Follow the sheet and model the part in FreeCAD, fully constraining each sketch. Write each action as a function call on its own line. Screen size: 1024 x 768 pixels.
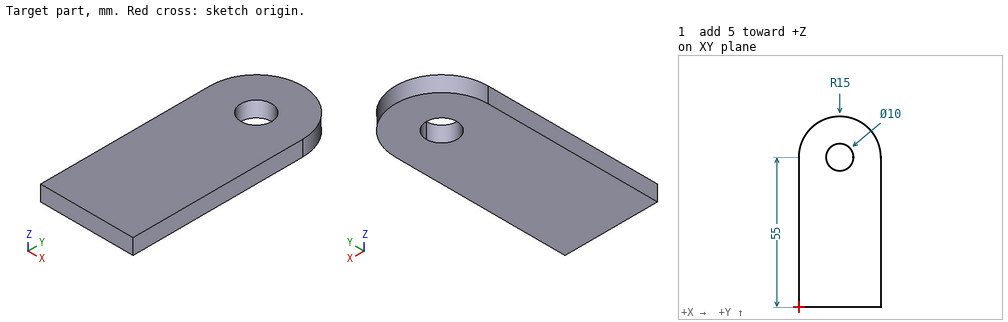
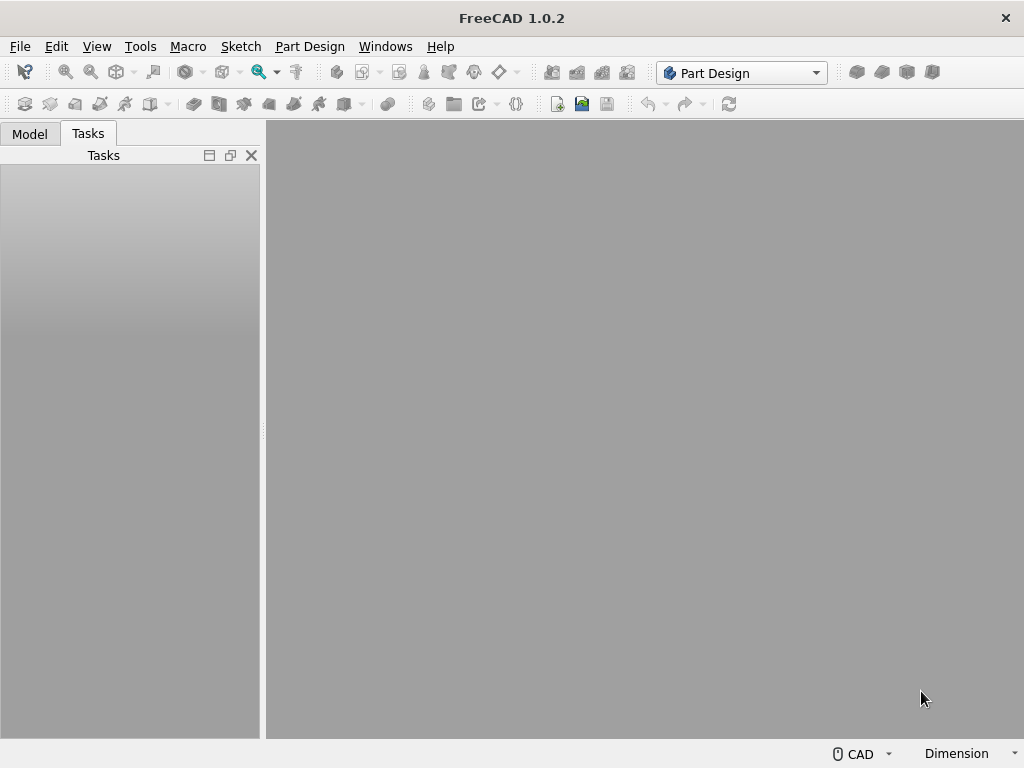
click(557, 104)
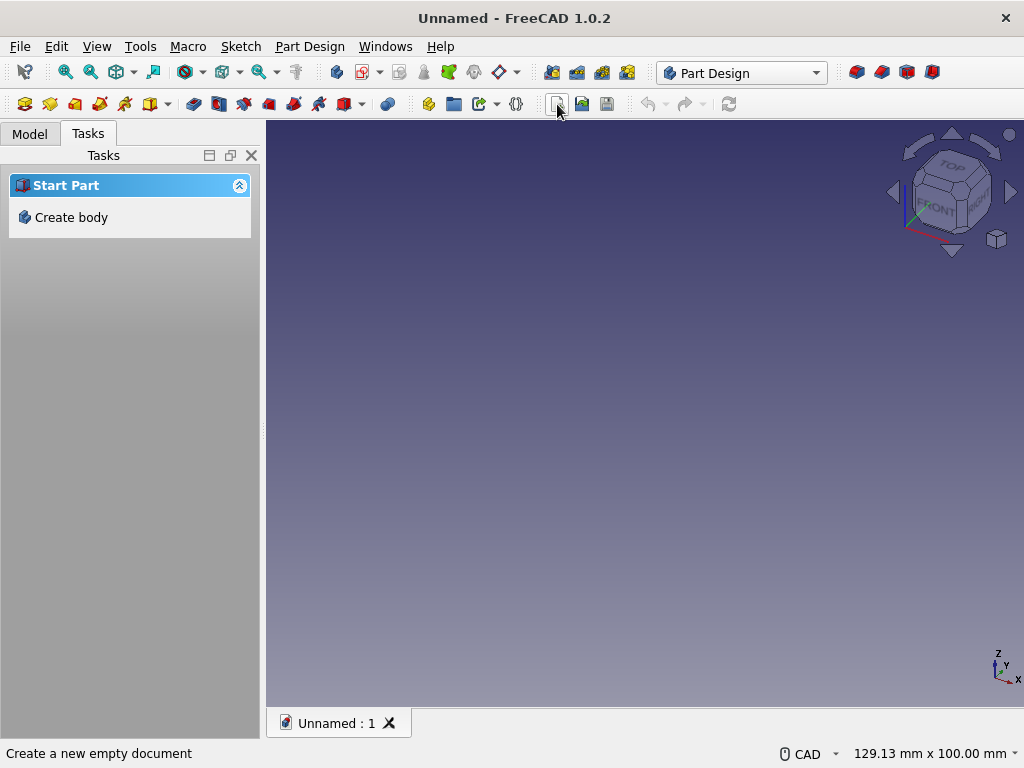
click(362, 72)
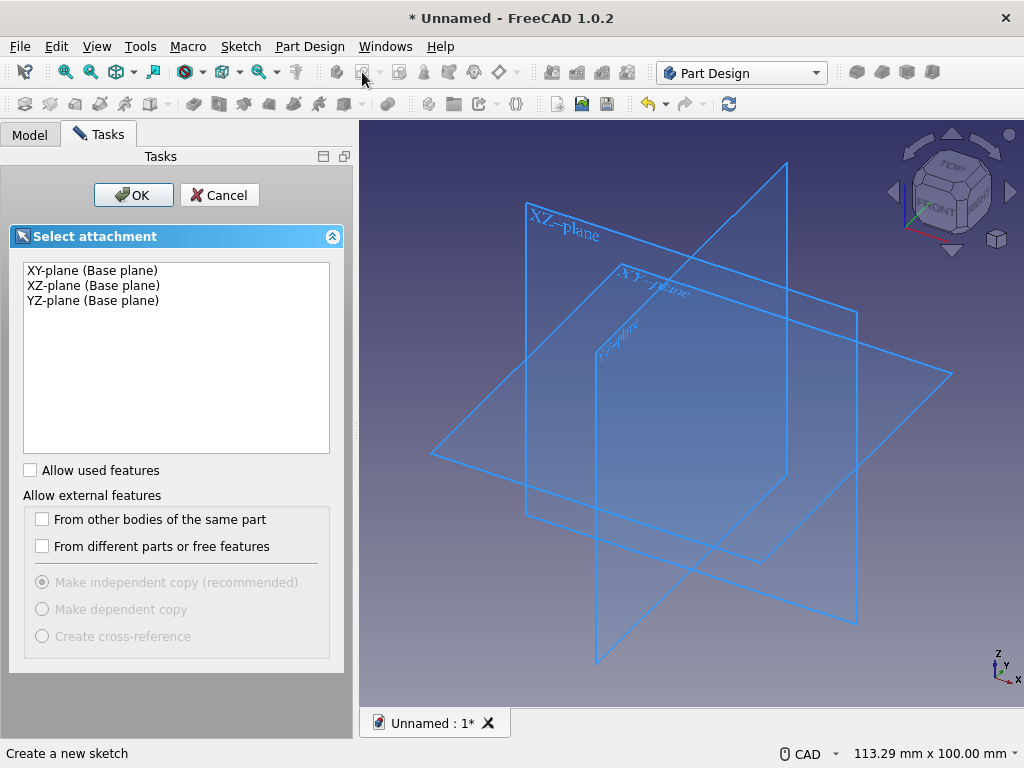
click(84, 270)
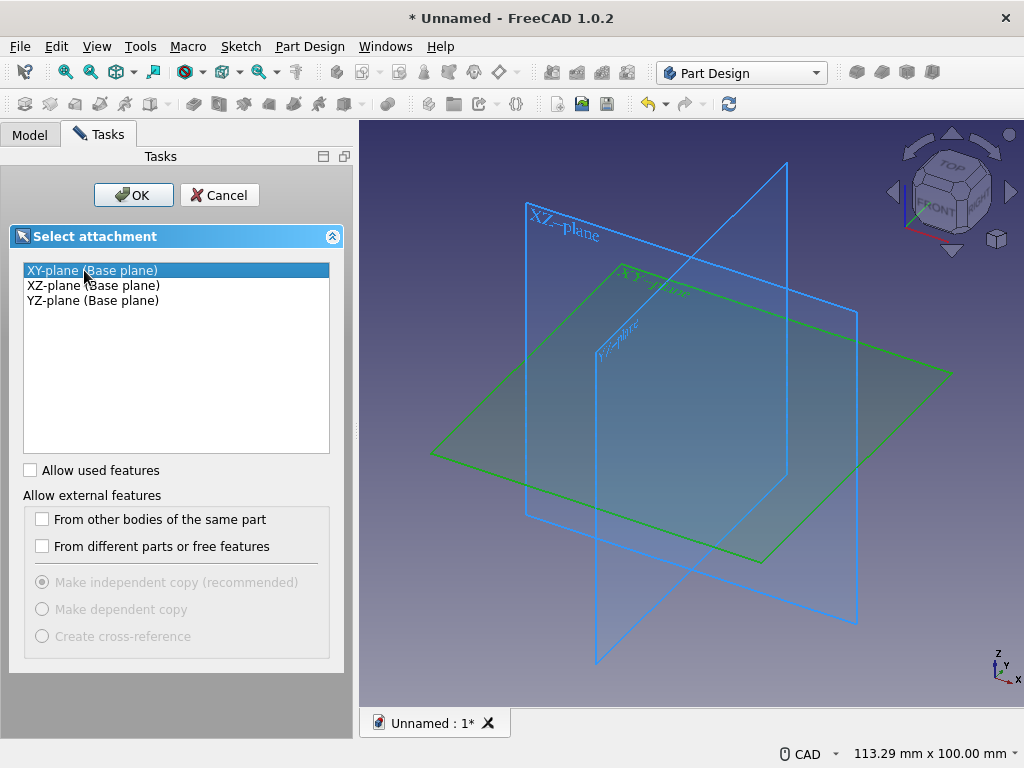
click(134, 195)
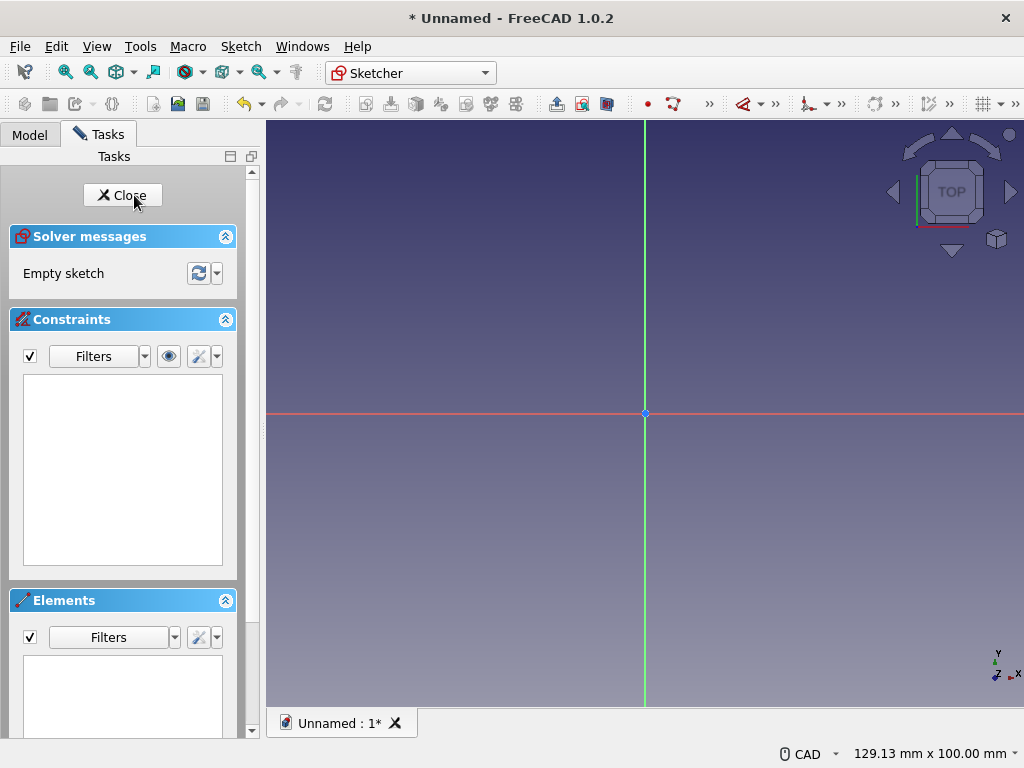
scroll(294, 679, down, 2)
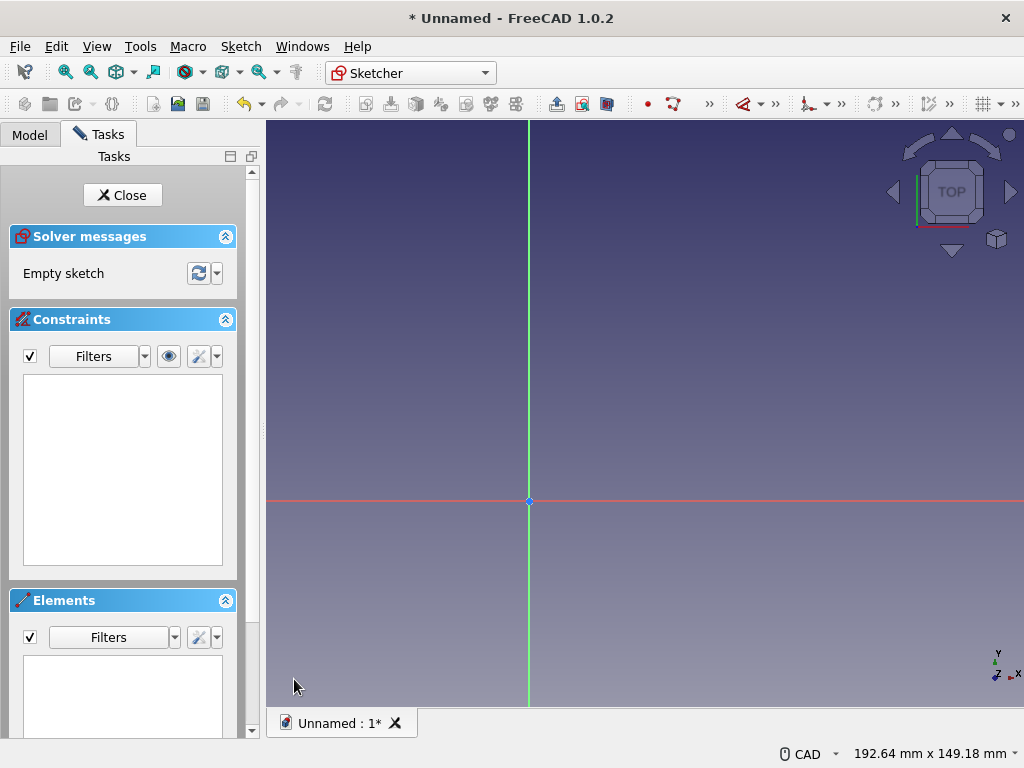
scroll(612, 262, up, 2)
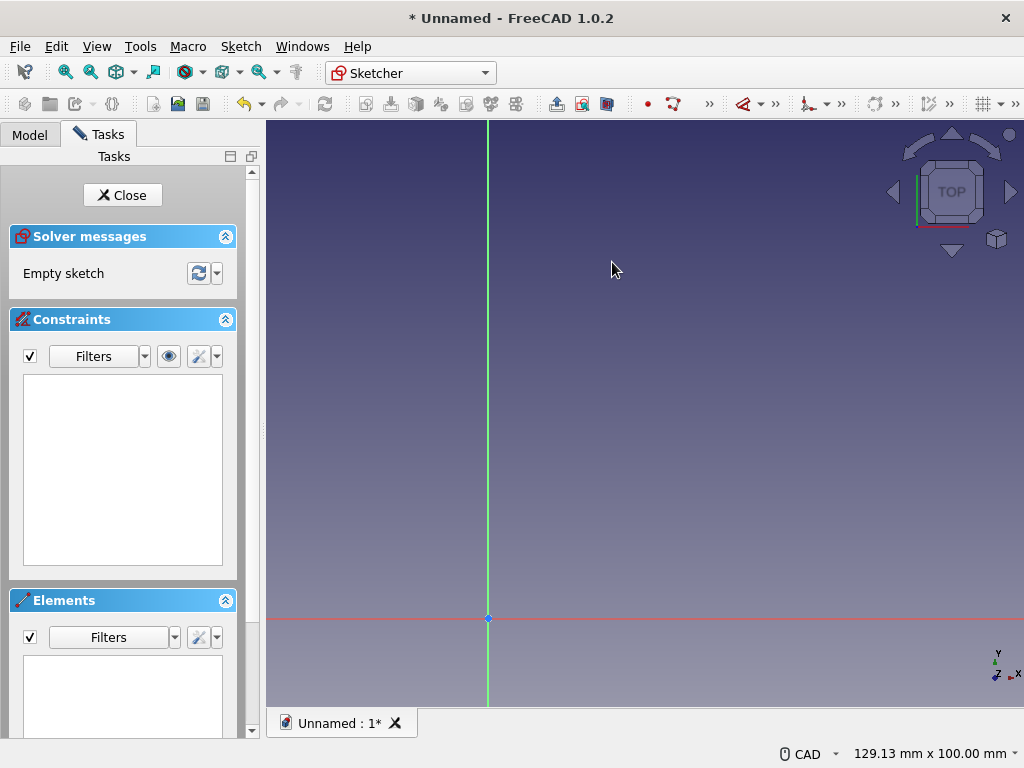
click(673, 104)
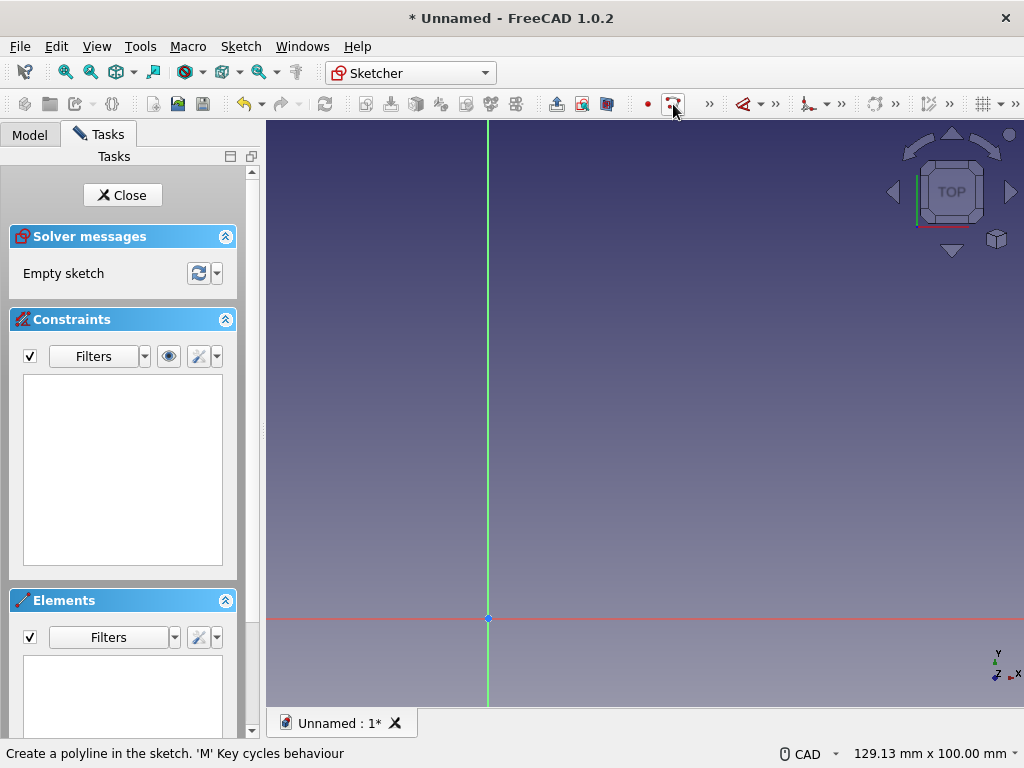
click(488, 296)
click(488, 619)
click(664, 610)
click(664, 296)
right_click(664, 296)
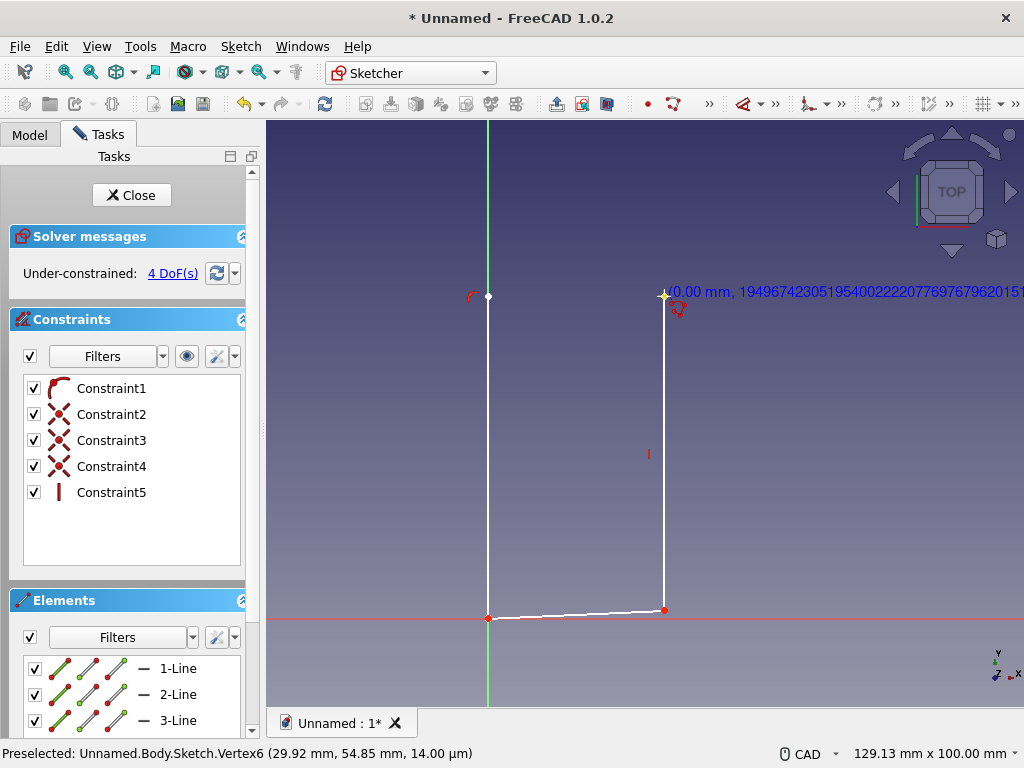
key(g)
key(3)
key(a)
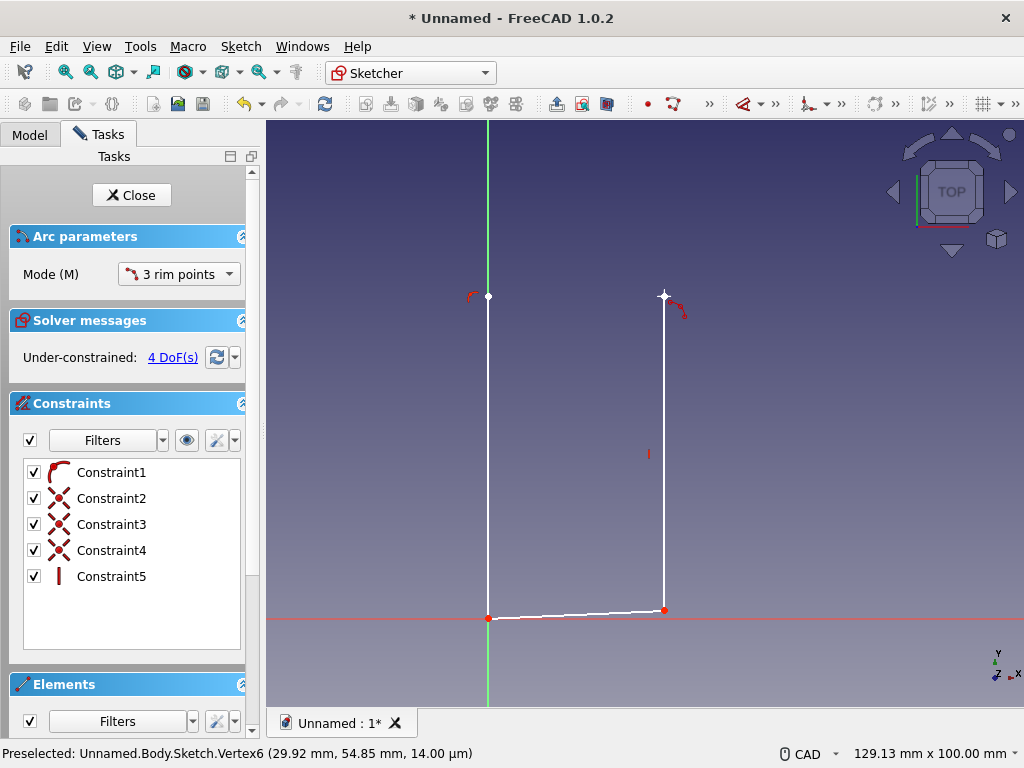
click(664, 297)
click(488, 297)
click(576, 208)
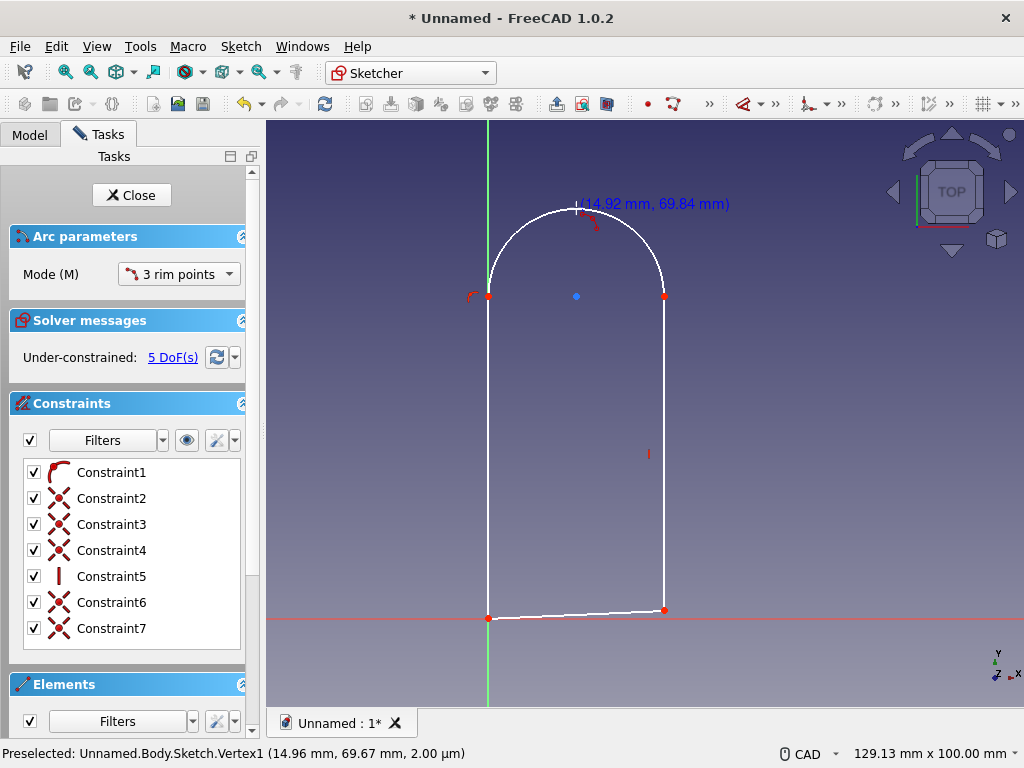
key(g)
key(c)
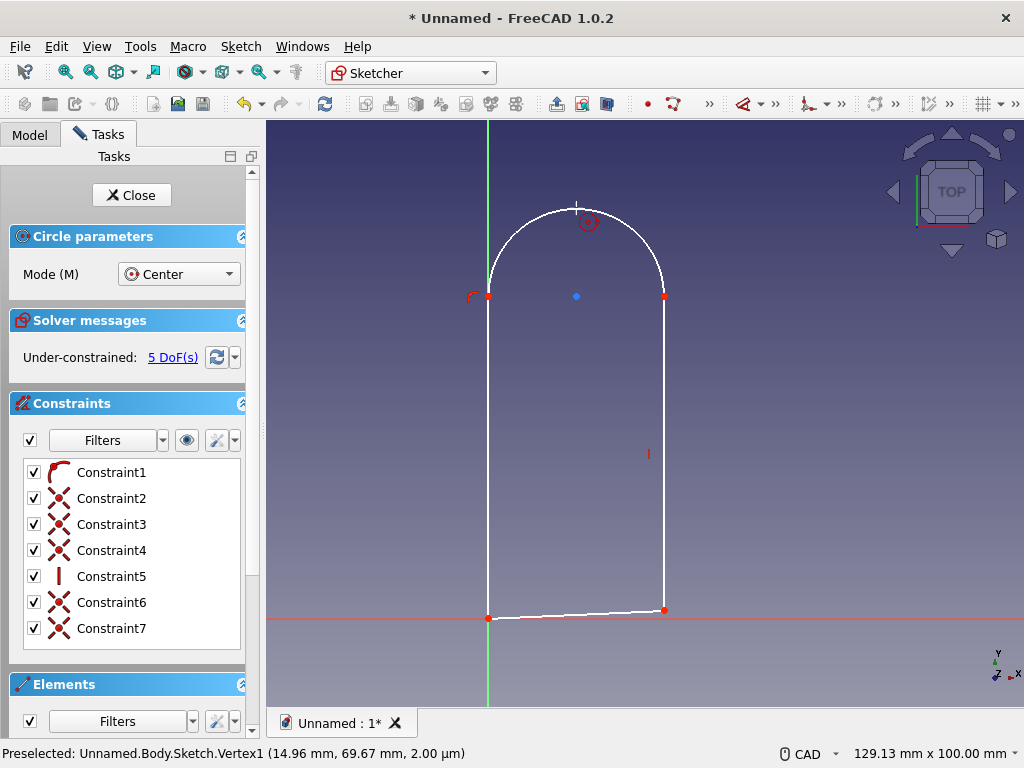
click(576, 296)
click(597, 275)
key(Escape)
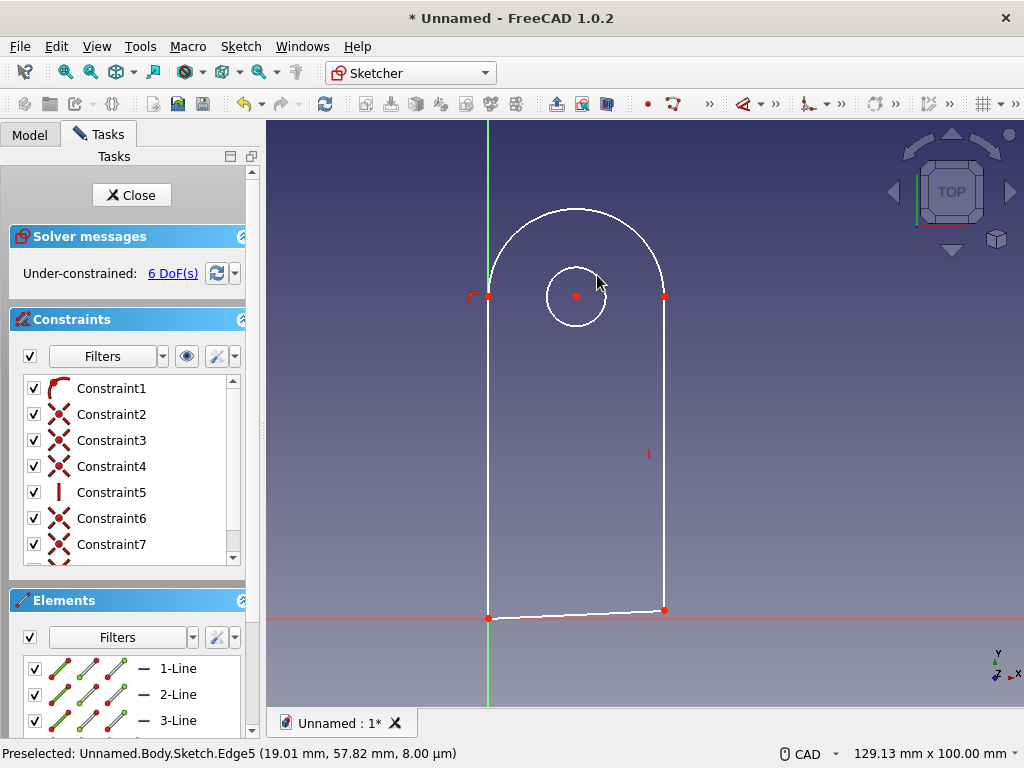
click(488, 394)